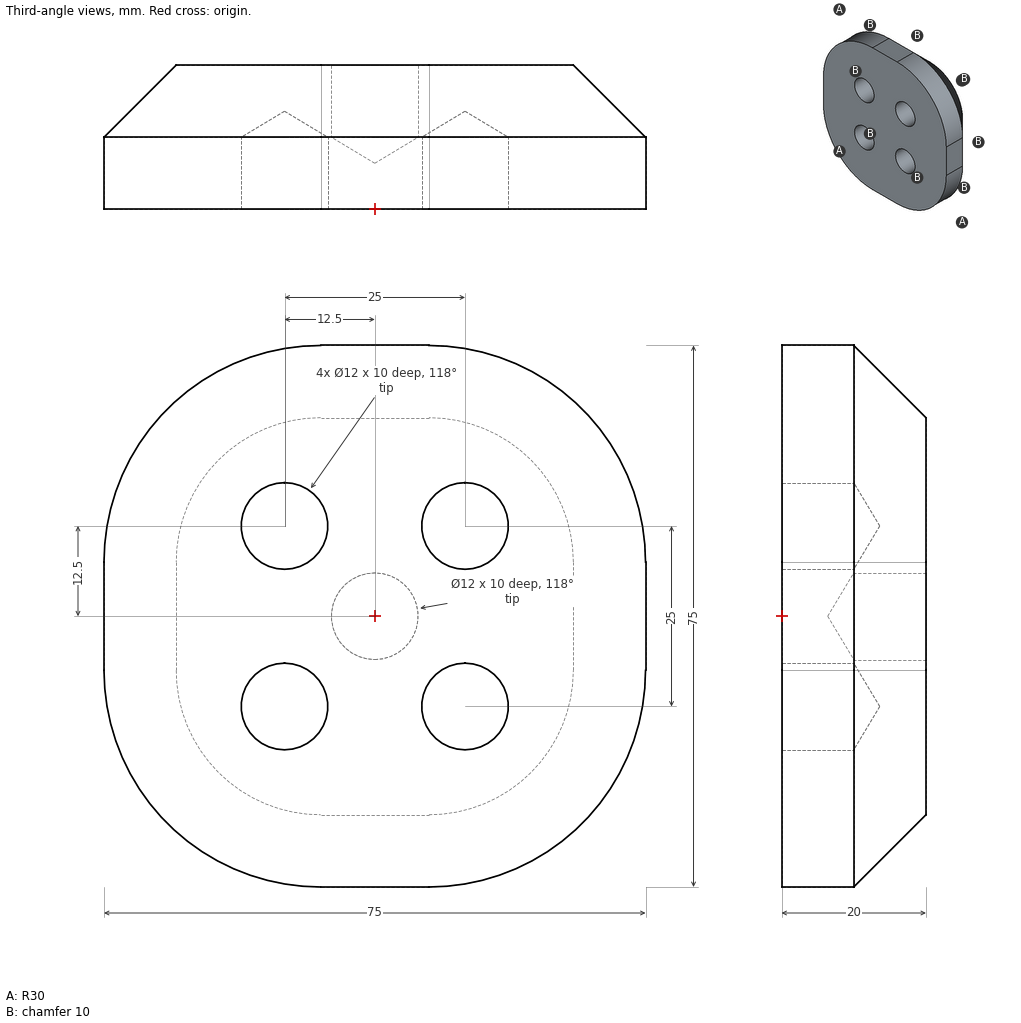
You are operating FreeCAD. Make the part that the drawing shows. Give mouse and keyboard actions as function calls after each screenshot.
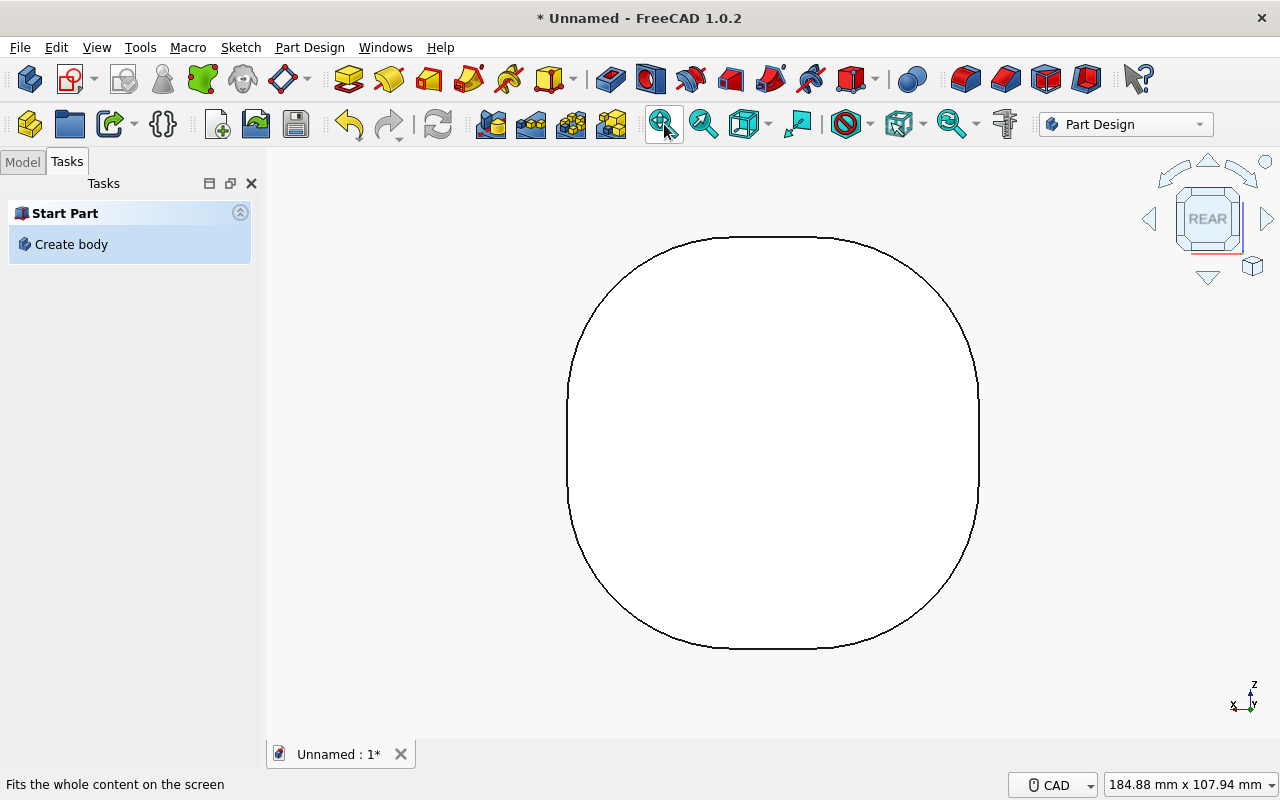
click(773, 442)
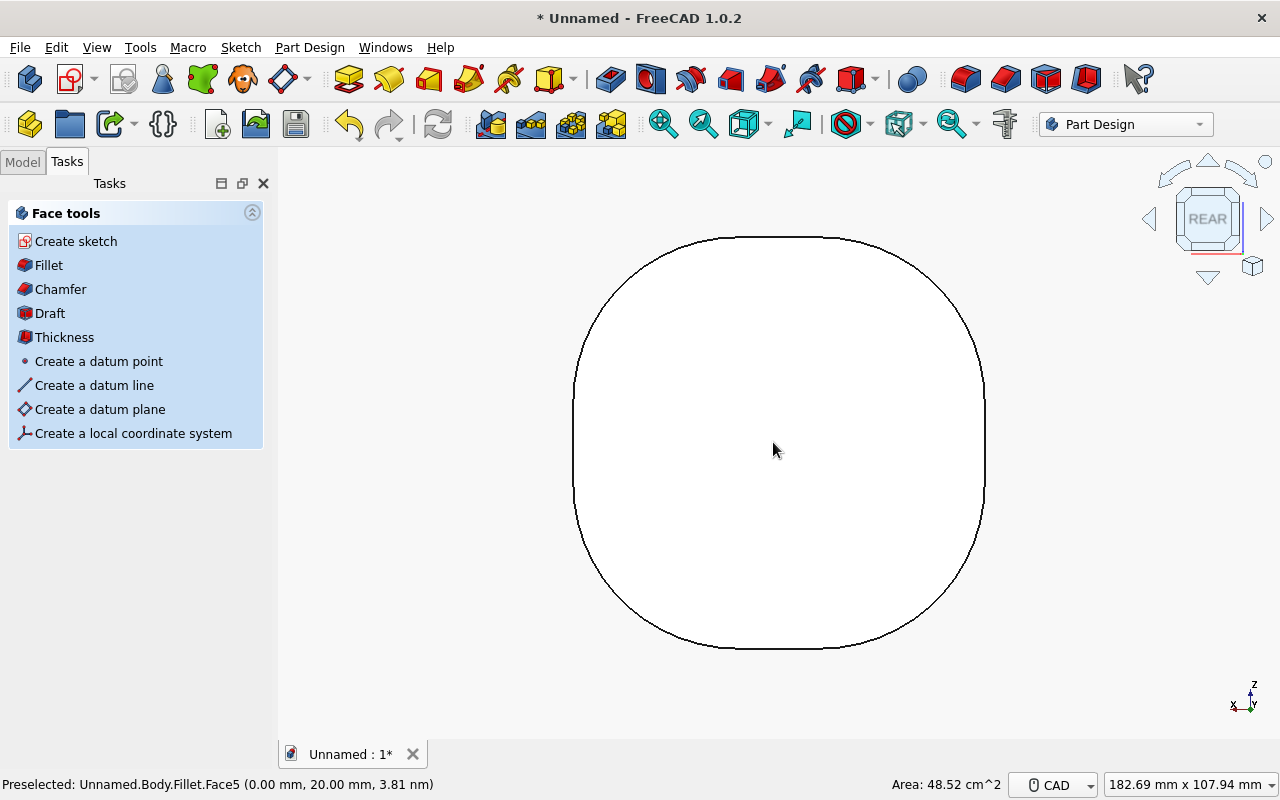
click(1006, 80)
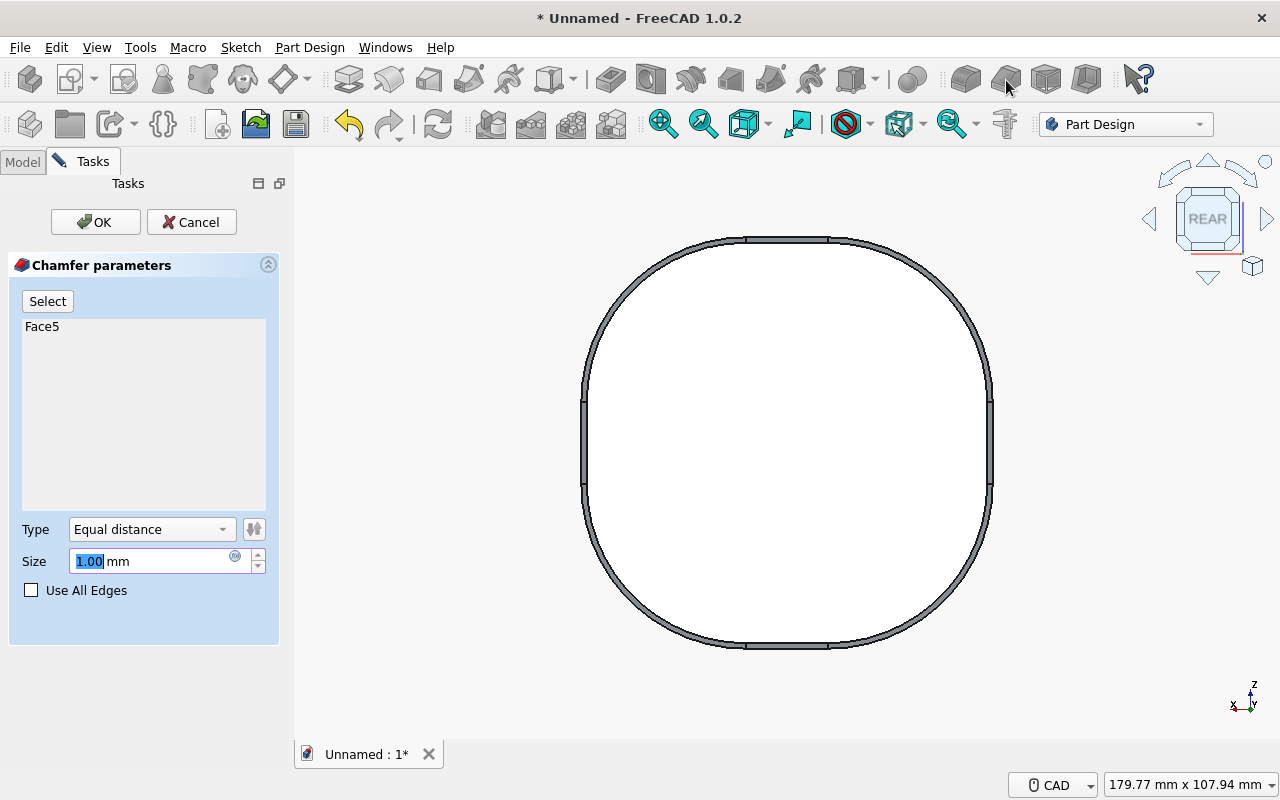
text(10)
key(Tab)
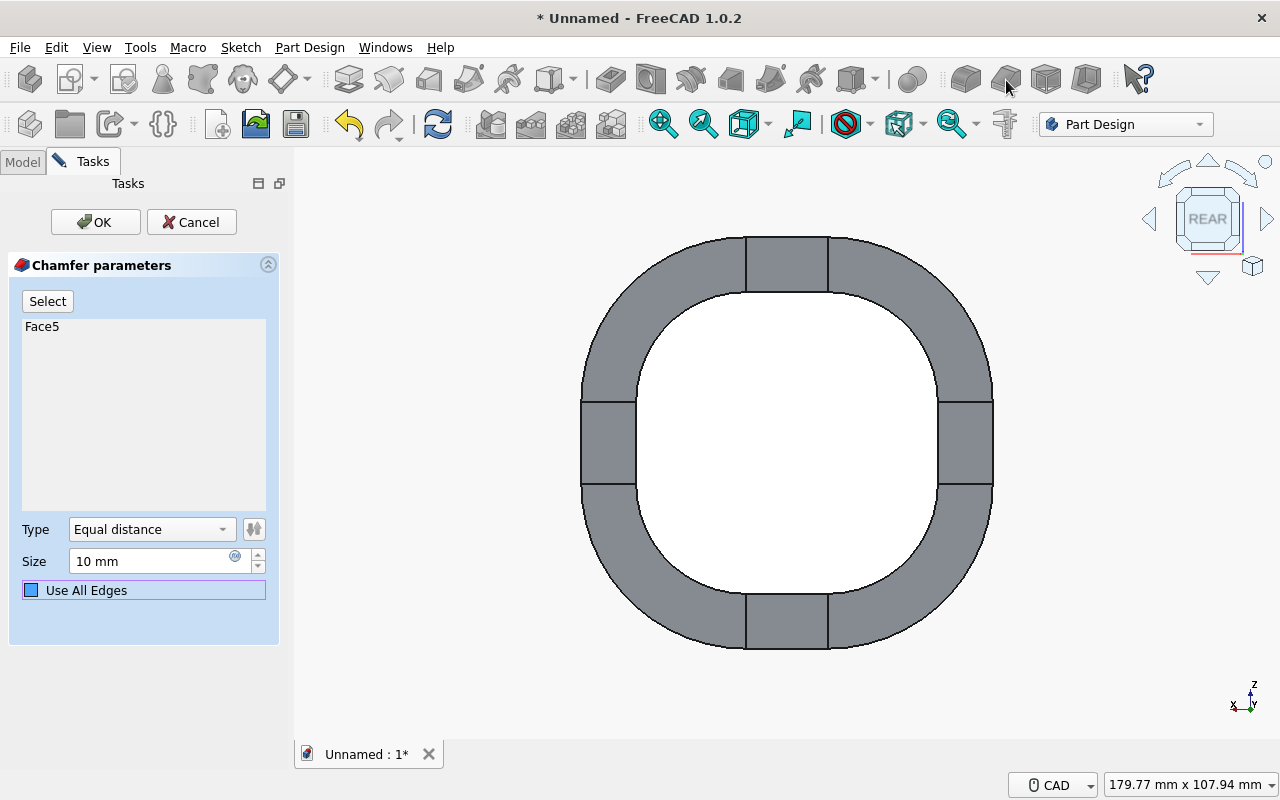
click(96, 222)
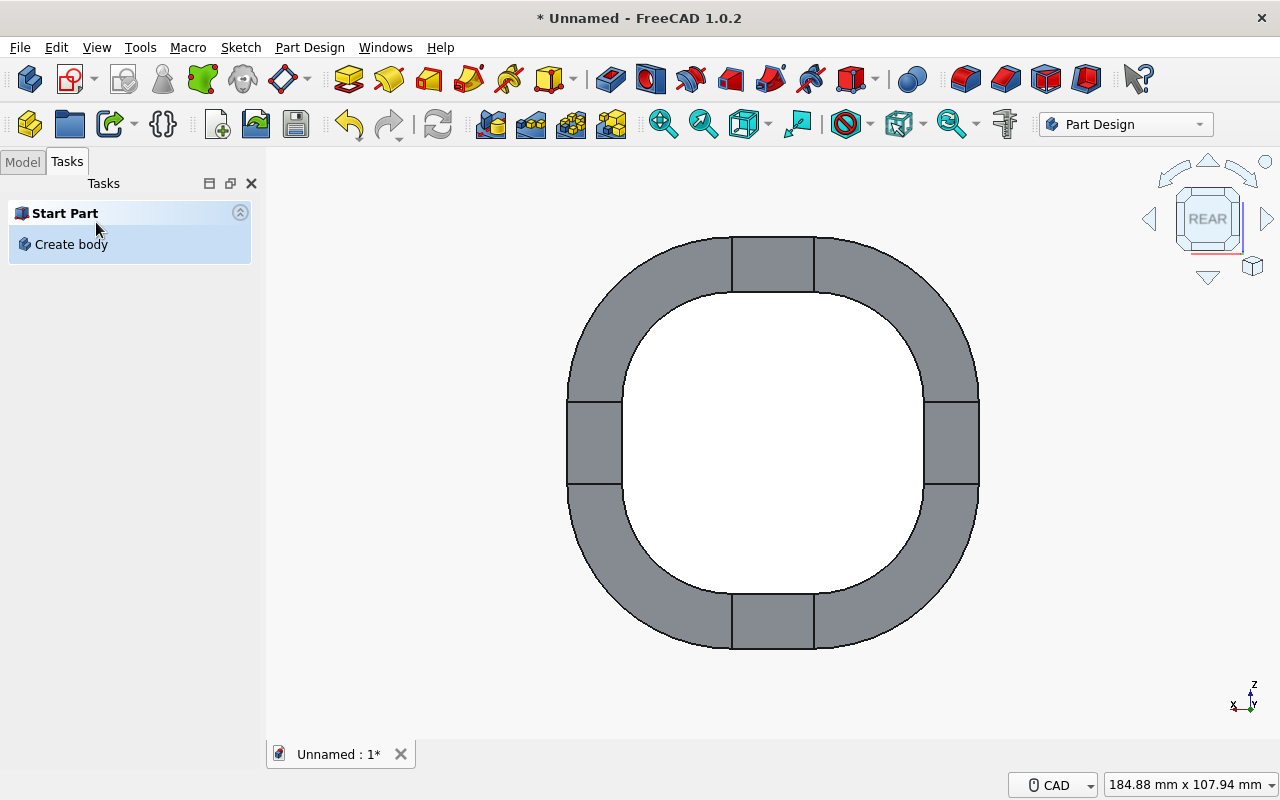
click(773, 442)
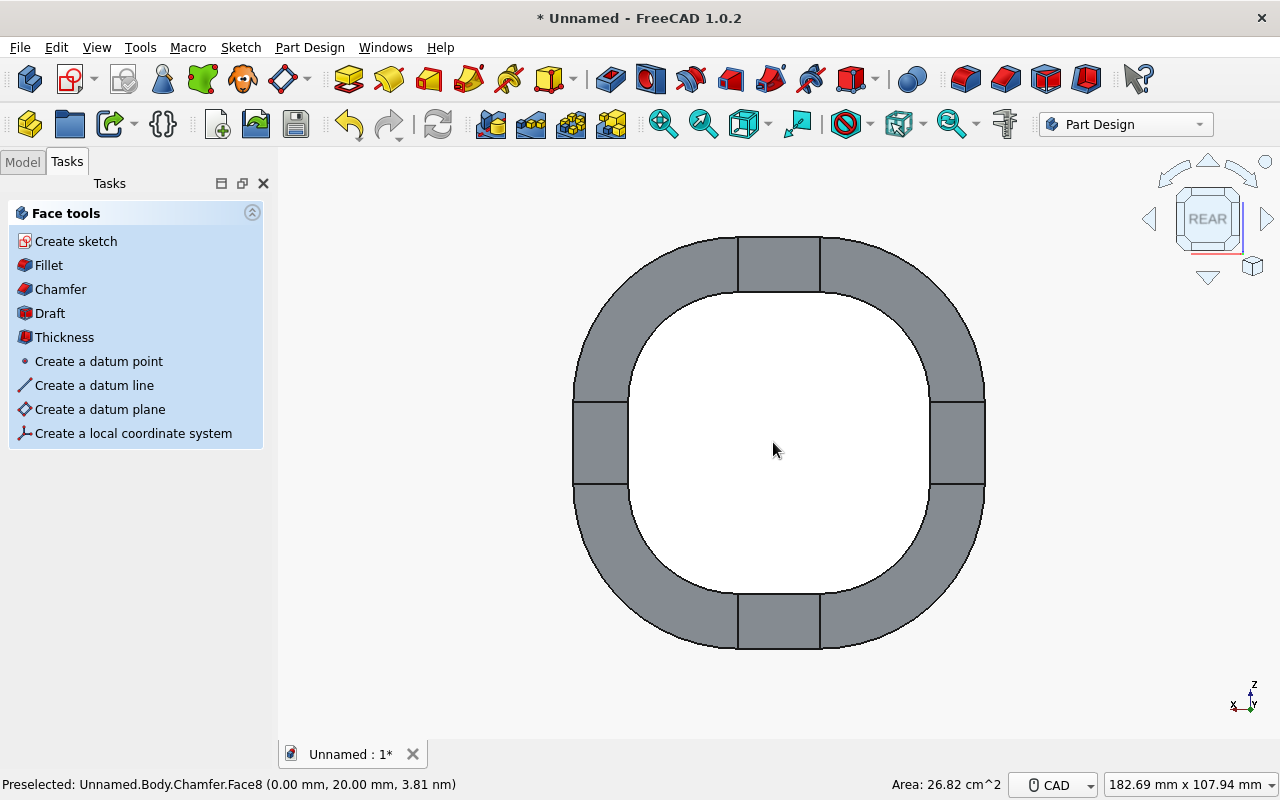
click(70, 80)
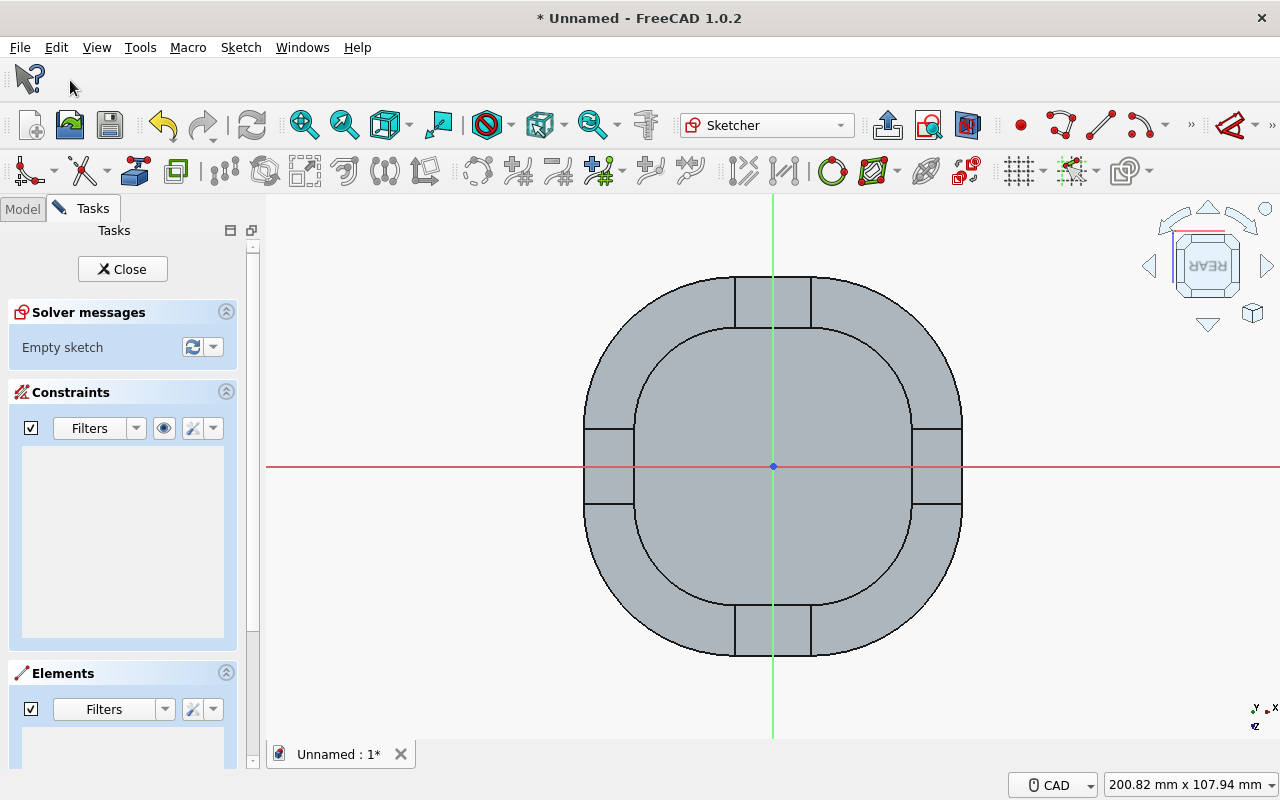
scroll(787, 466, up, 9)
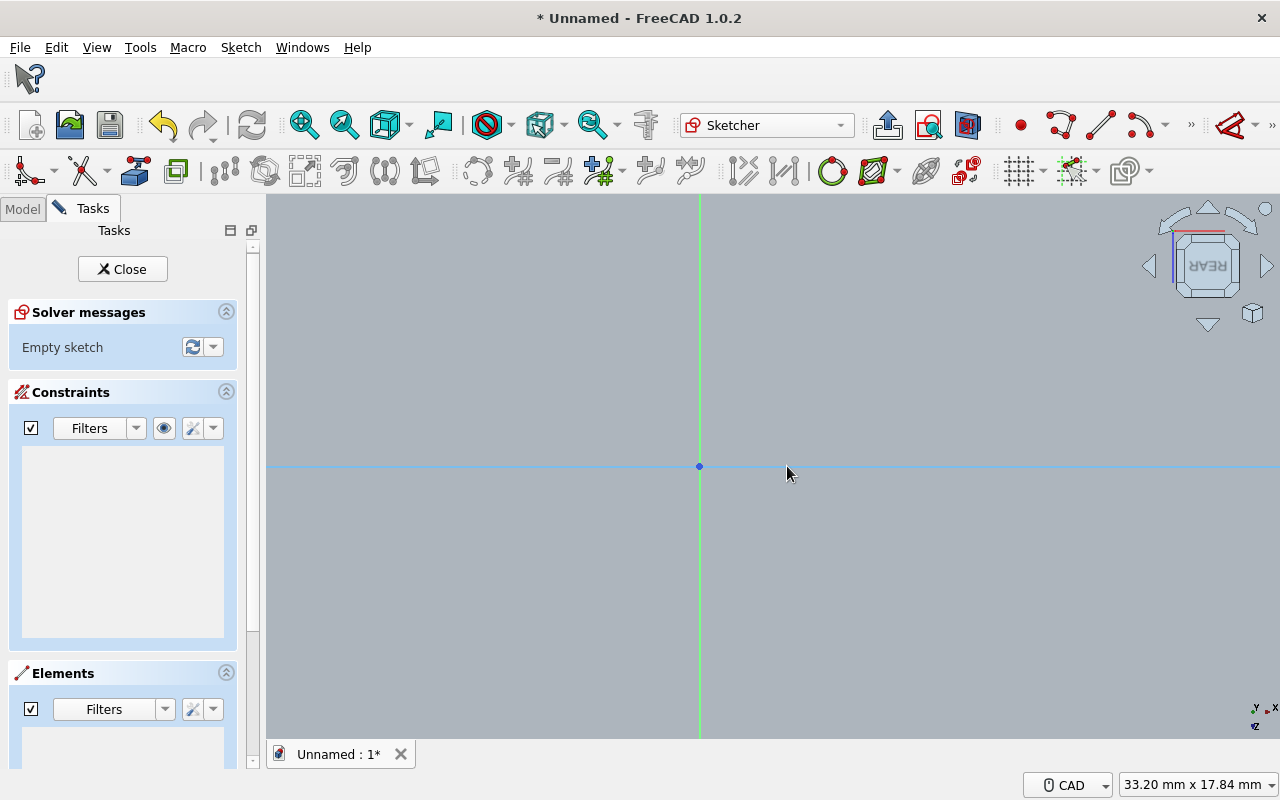
key(g)
key(c)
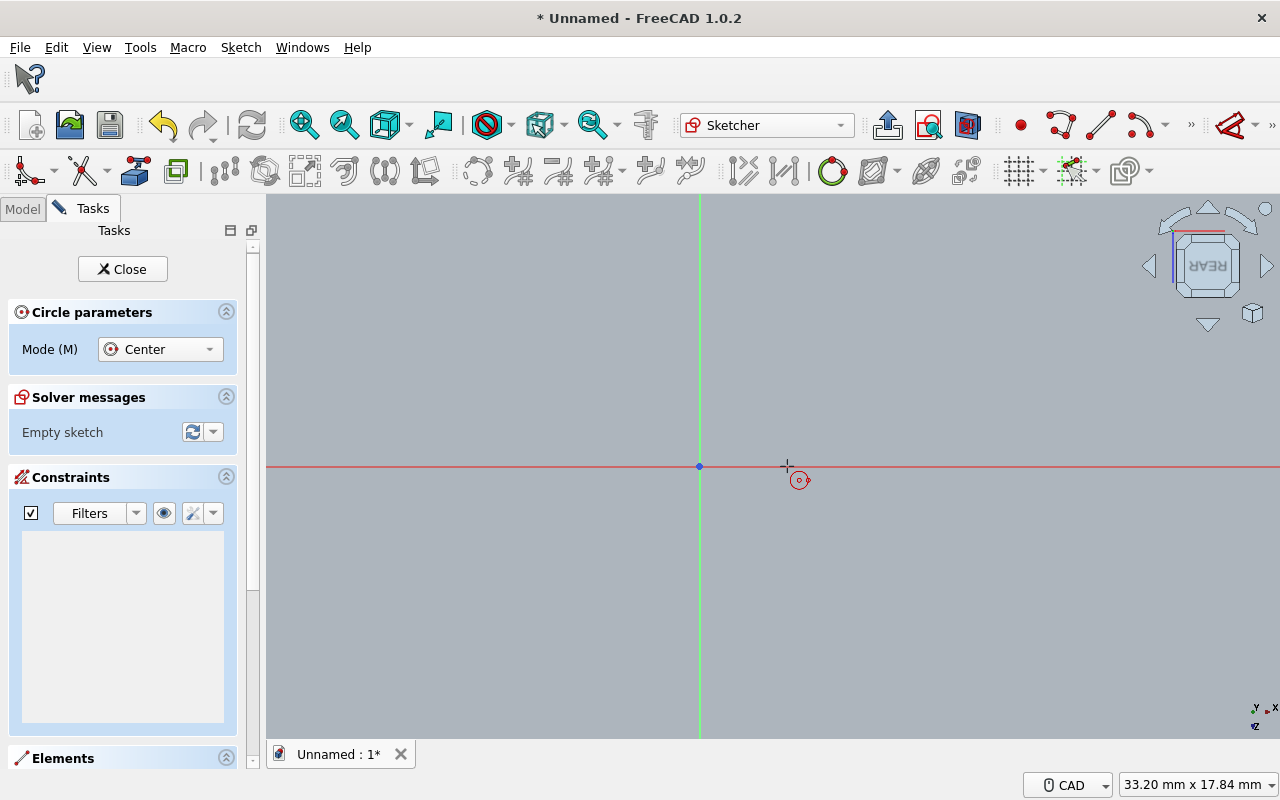
click(700, 466)
click(829, 337)
key(Escape)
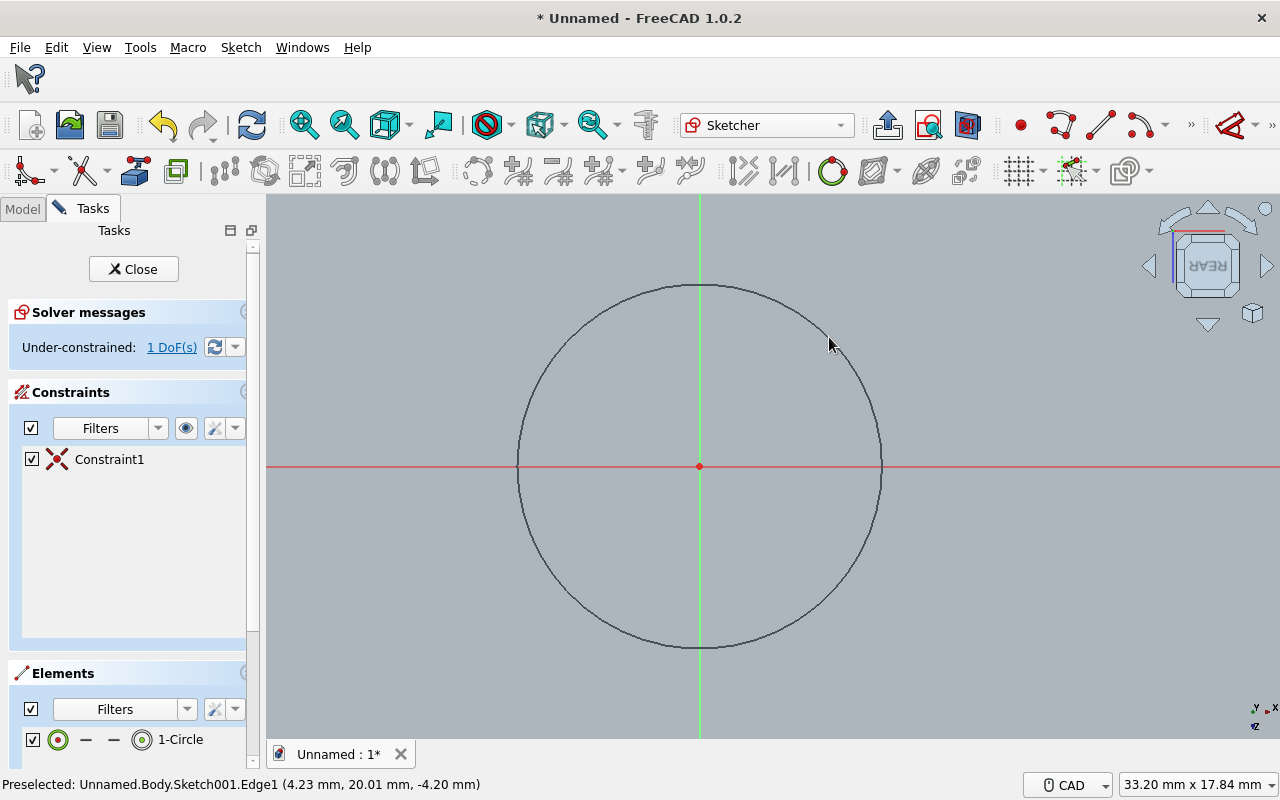
click(1230, 126)